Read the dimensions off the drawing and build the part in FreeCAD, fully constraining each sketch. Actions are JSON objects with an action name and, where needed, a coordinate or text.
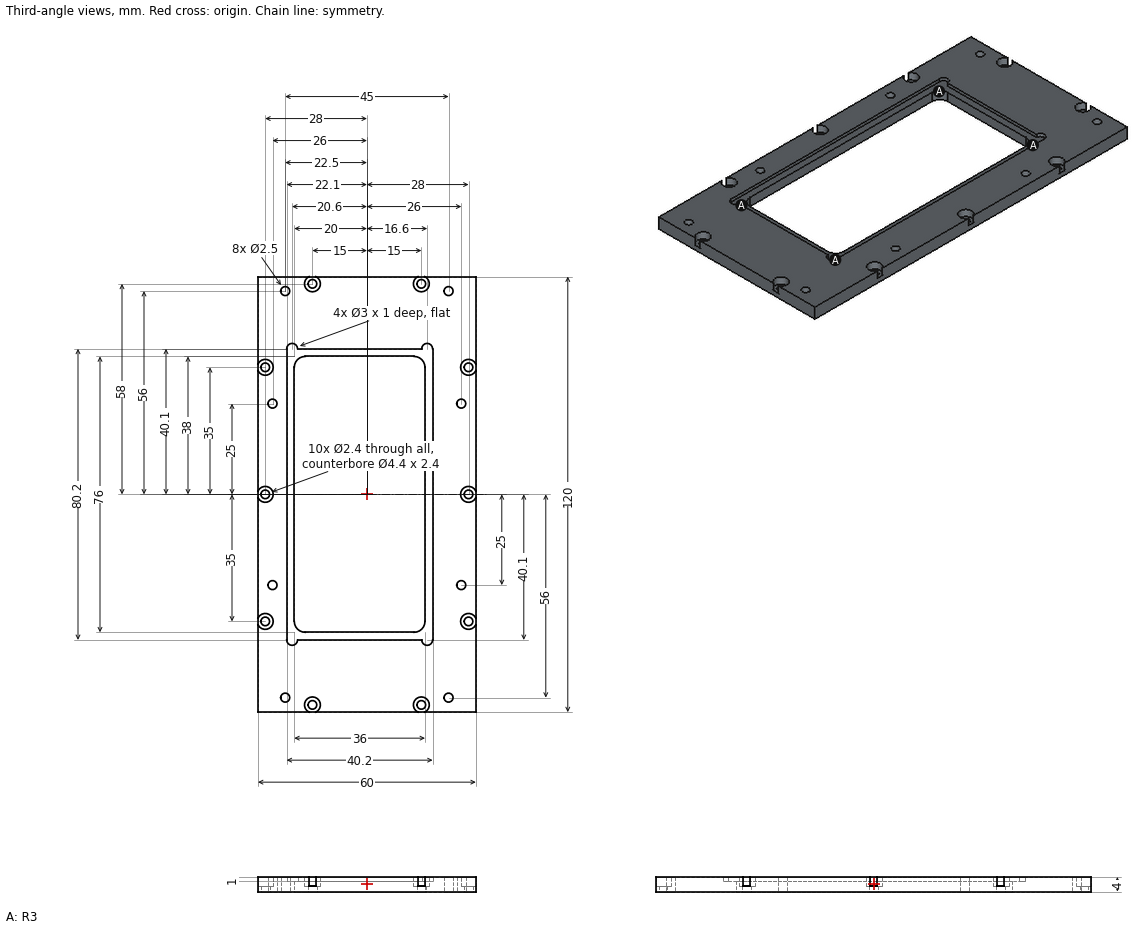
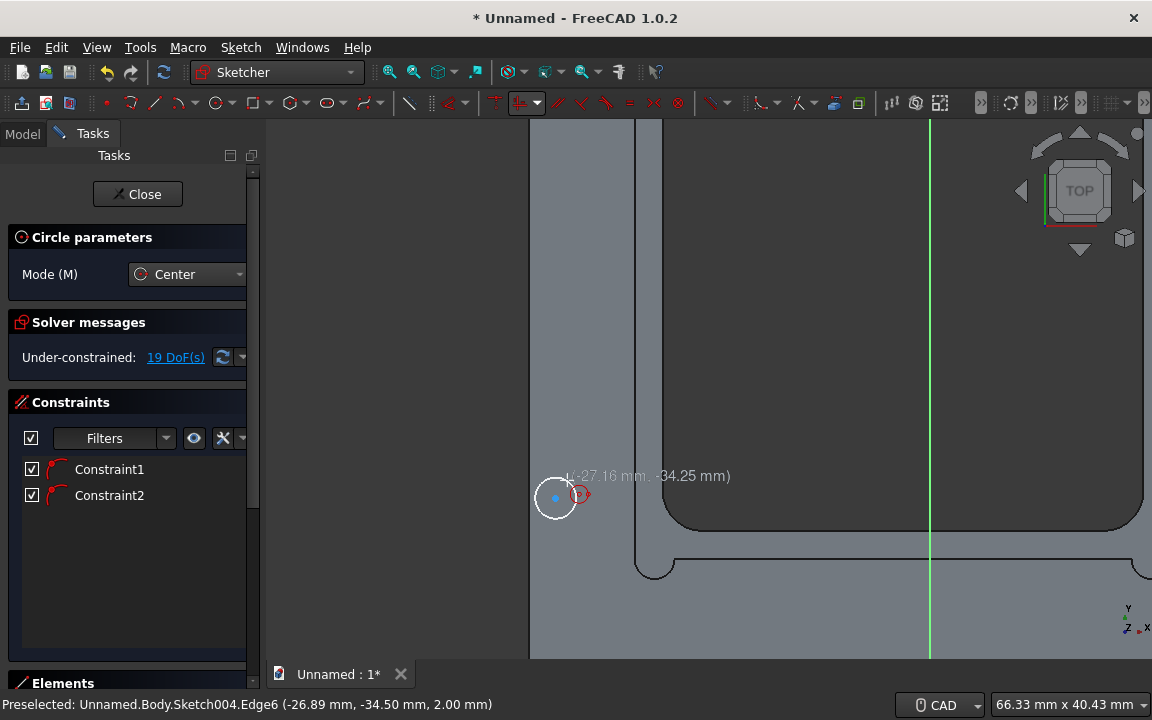
{"action": "scroll", "coordinate": [567, 481], "scroll_direction": "down", "scroll_amount": 8}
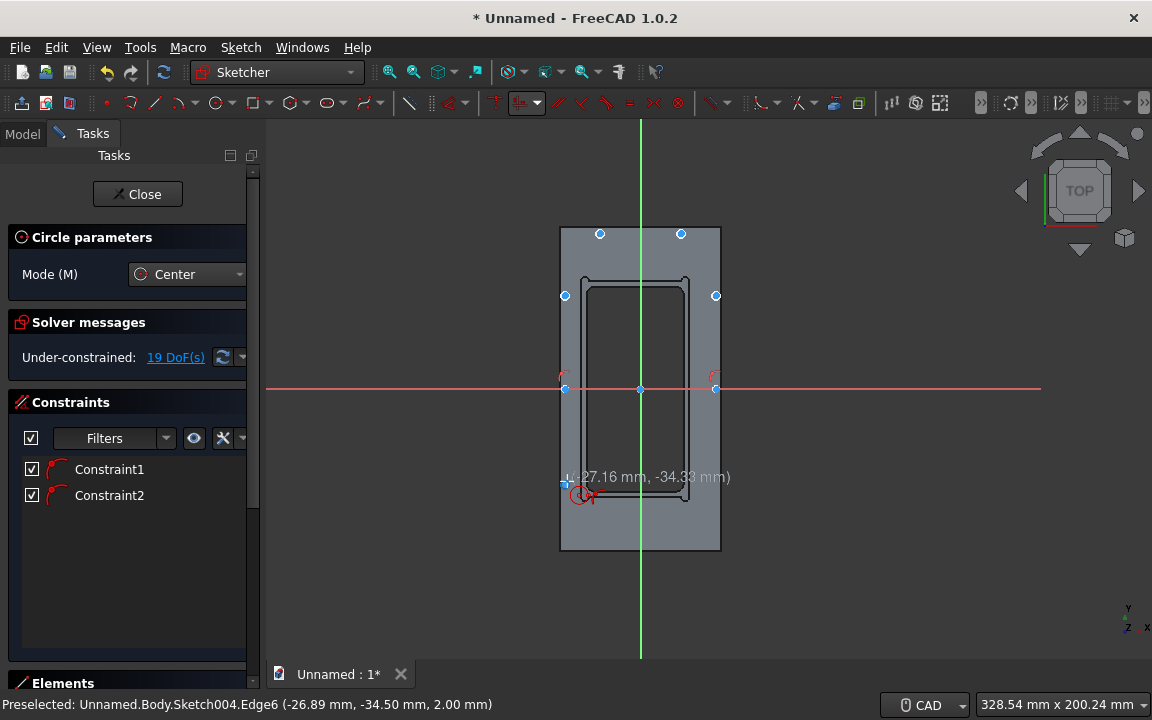
{"action": "scroll", "coordinate": [716, 484], "scroll_direction": "up", "scroll_amount": 10}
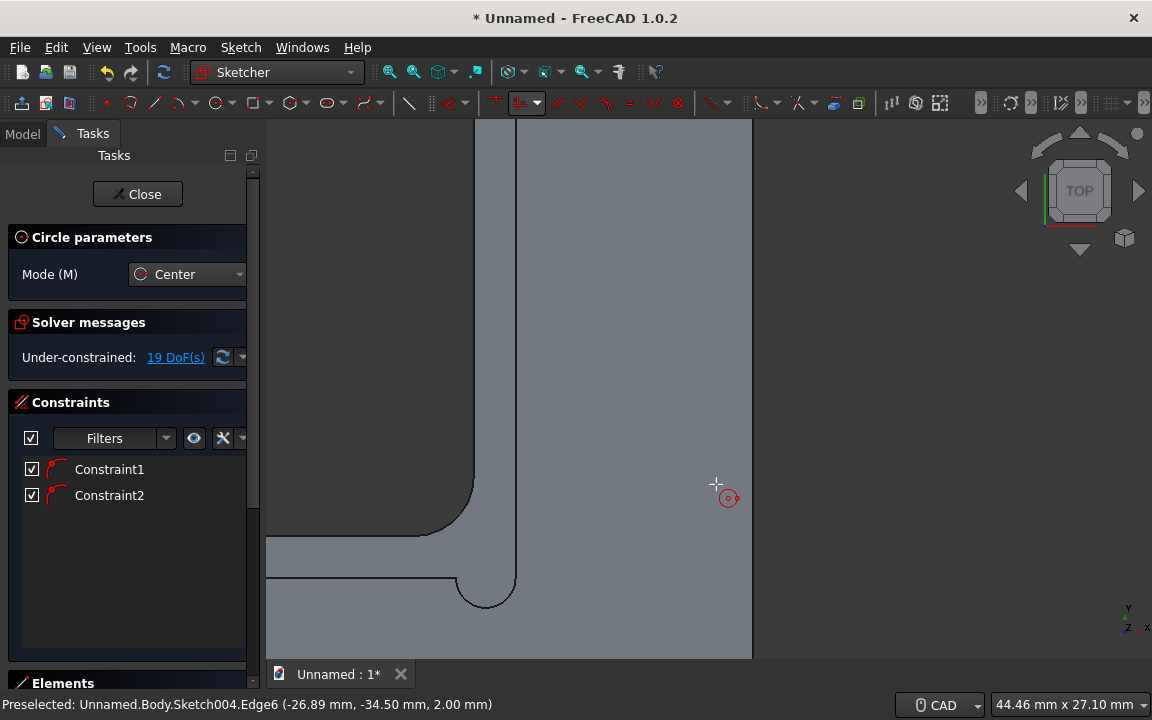
{"action": "scroll", "coordinate": [716, 484], "scroll_direction": "down", "scroll_amount": 10}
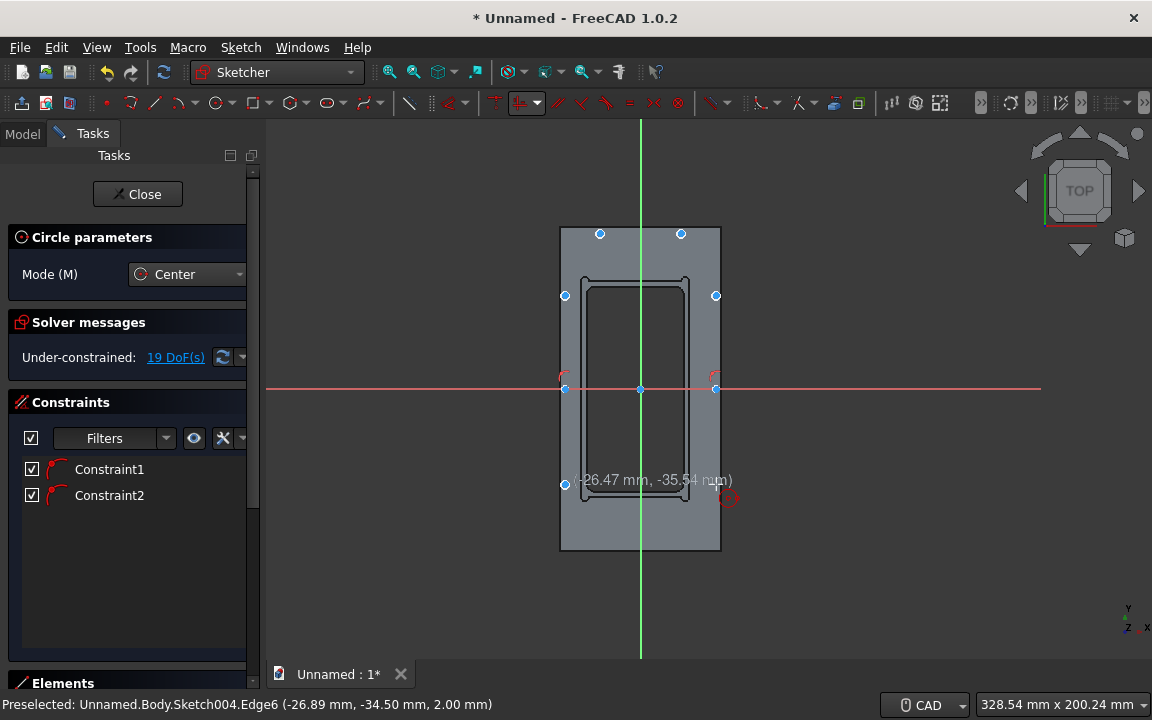
{"action": "left_click", "coordinate": [716, 484]}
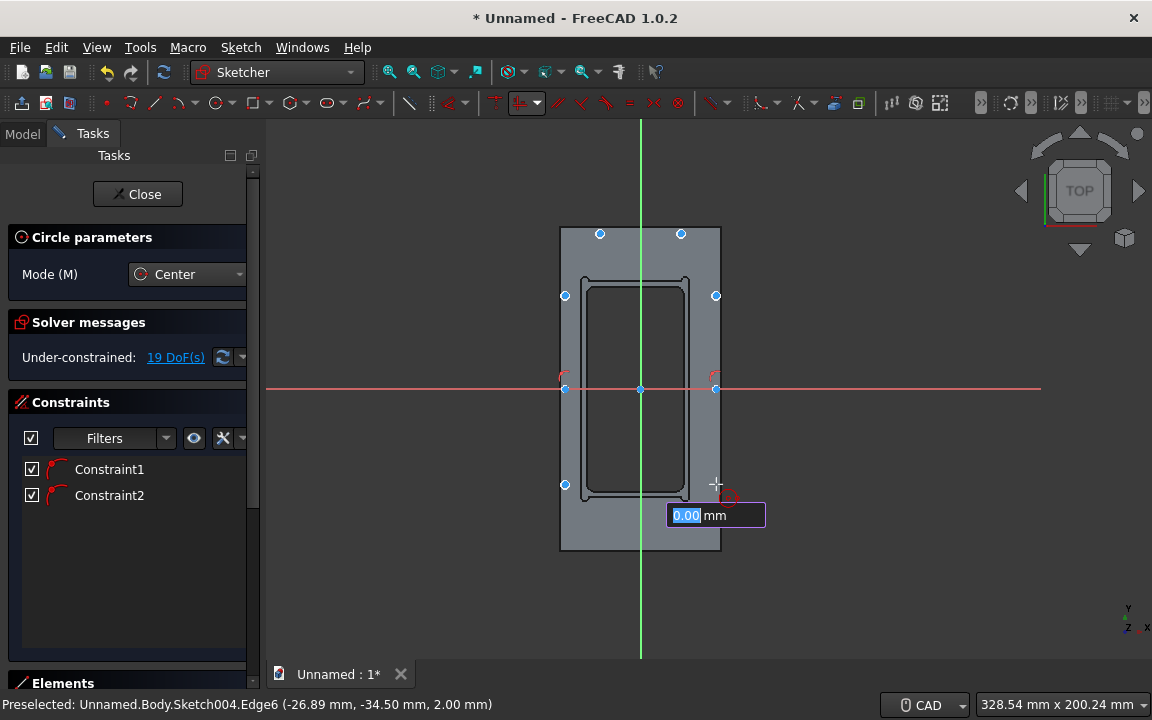
{"action": "scroll", "coordinate": [718, 481], "scroll_direction": "up", "scroll_amount": 8}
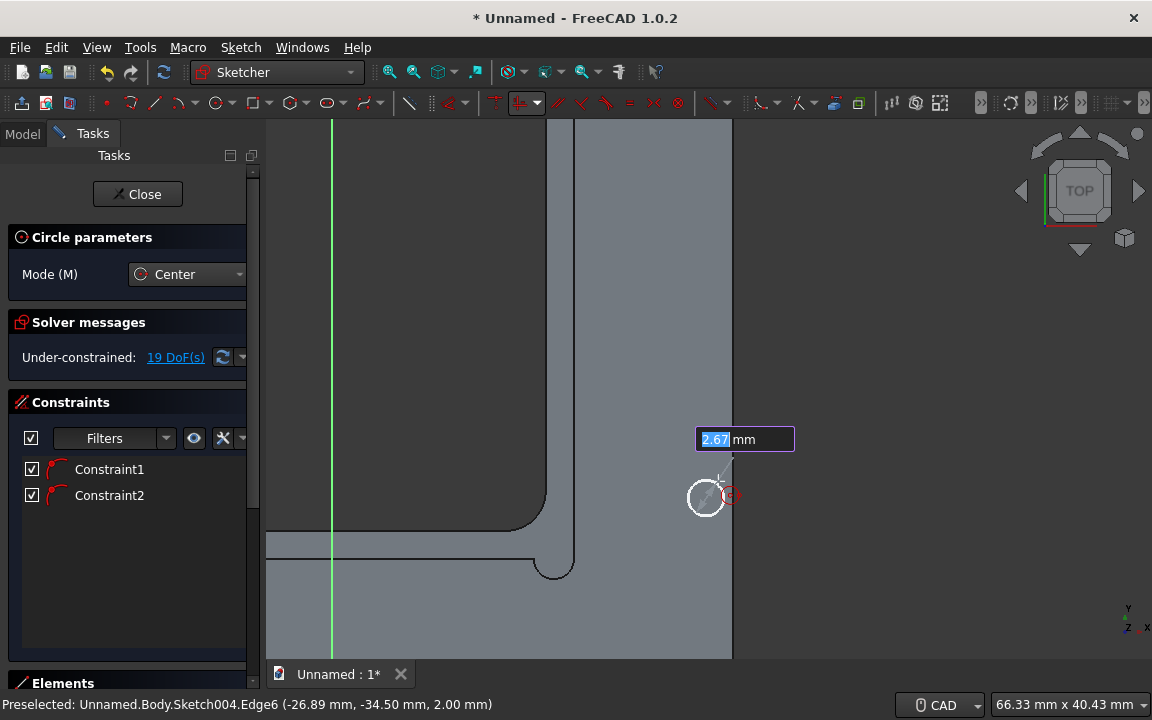
{"action": "left_click", "coordinate": [718, 480]}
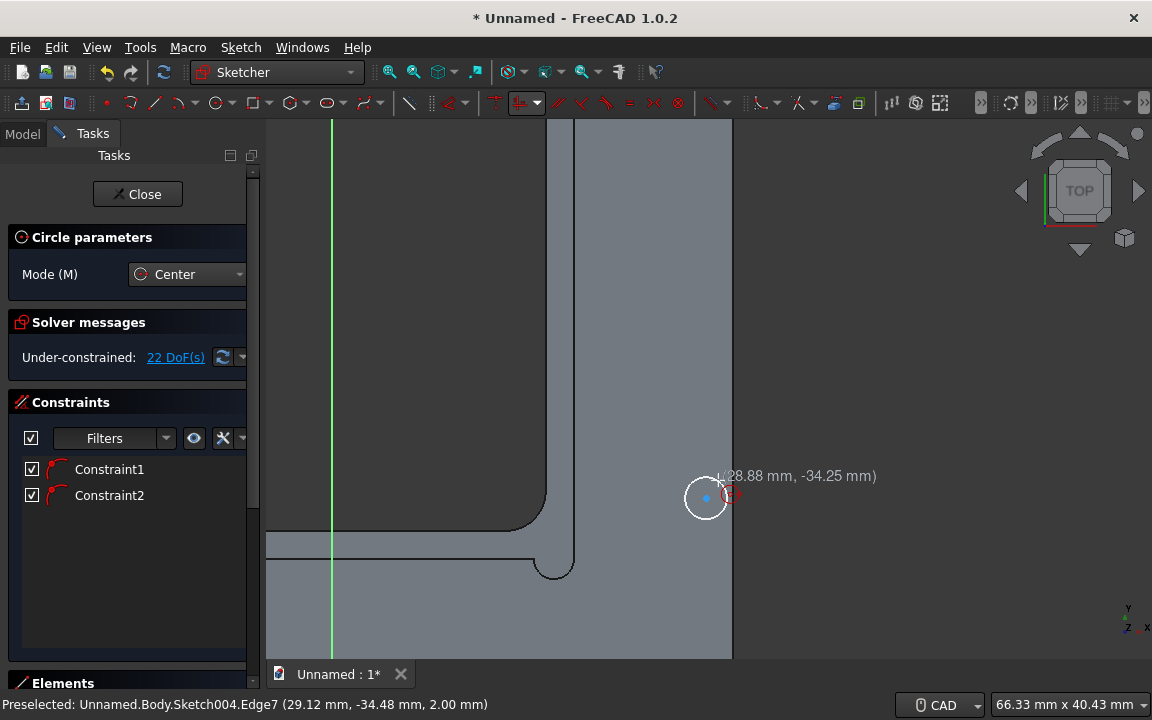
{"action": "scroll", "coordinate": [718, 481], "scroll_direction": "down", "scroll_amount": 8}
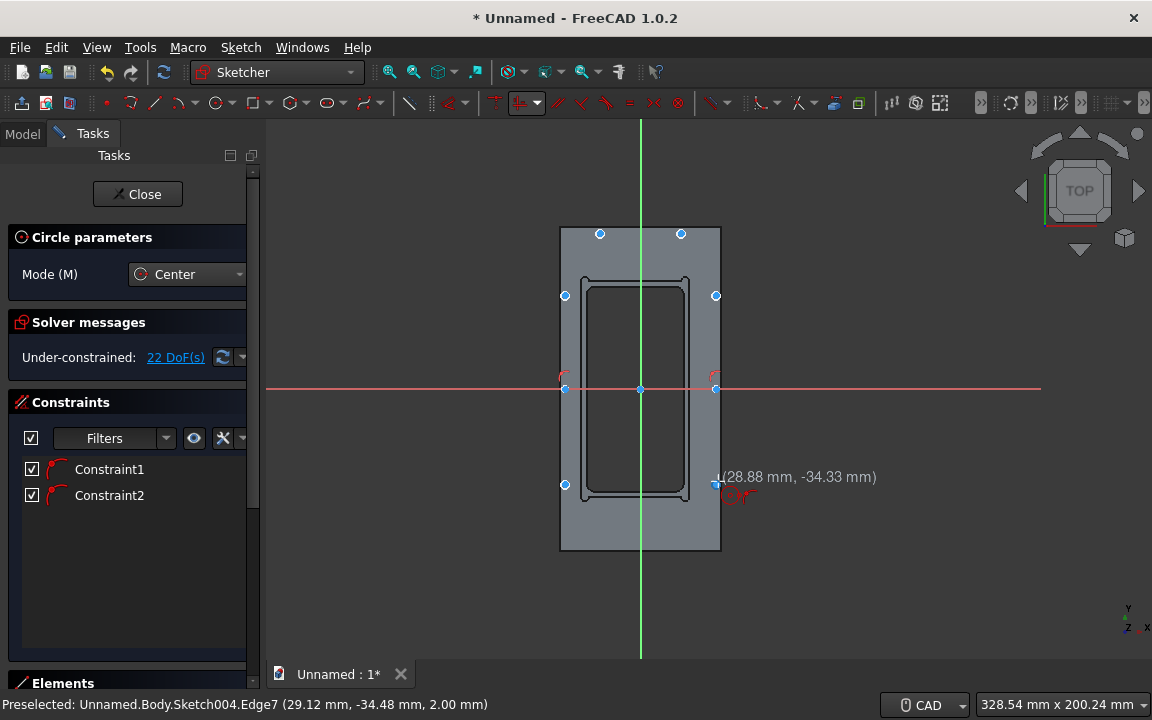
{"action": "scroll", "coordinate": [600, 546], "scroll_direction": "up", "scroll_amount": 10}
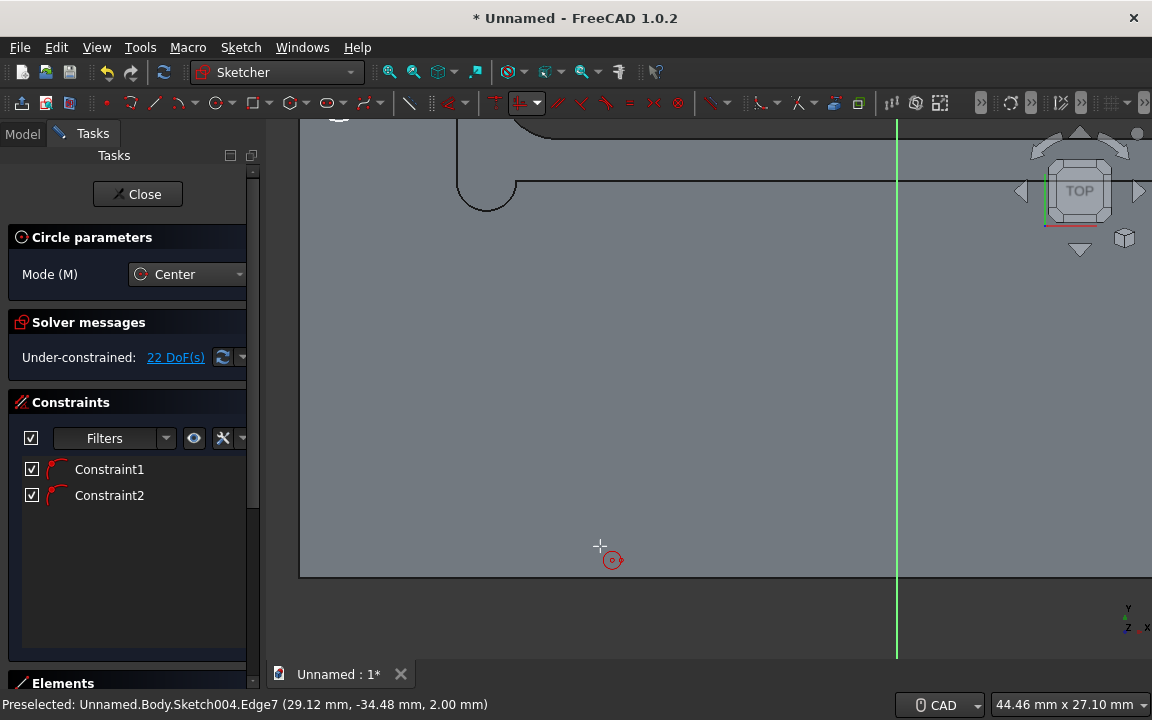
{"action": "scroll", "coordinate": [600, 547], "scroll_direction": "down", "scroll_amount": 10}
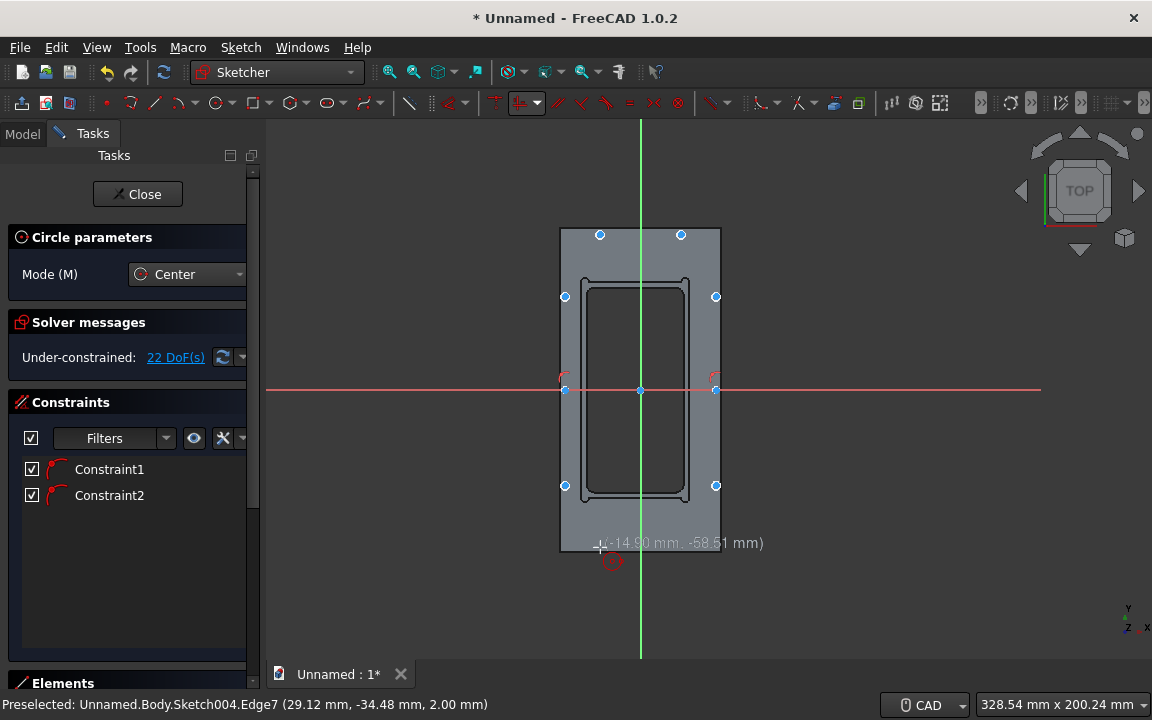
{"action": "left_click", "coordinate": [600, 546]}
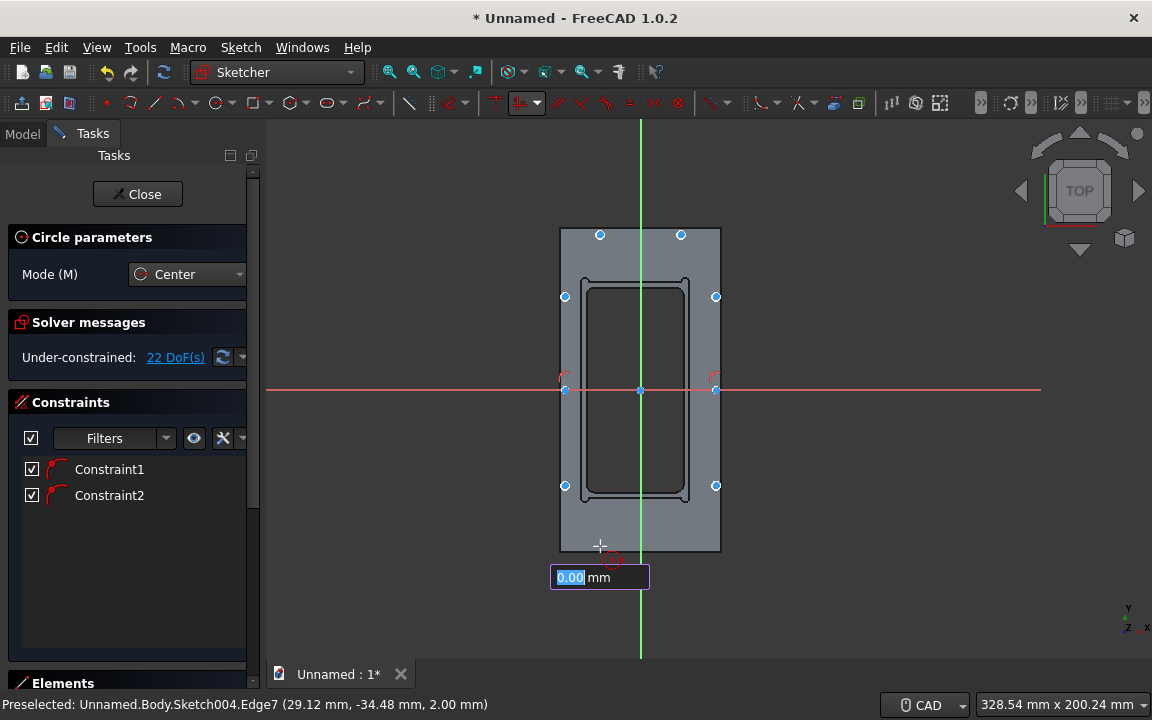
{"action": "scroll", "coordinate": [602, 544], "scroll_direction": "up", "scroll_amount": 8}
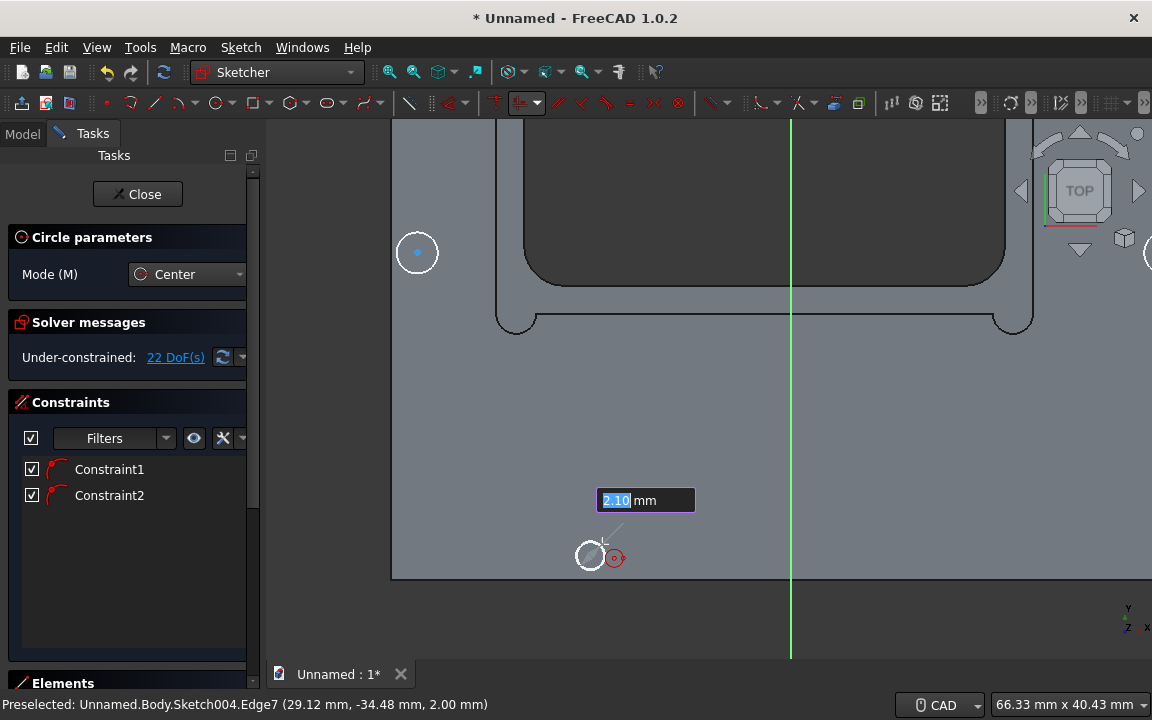
{"action": "left_click", "coordinate": [602, 542]}